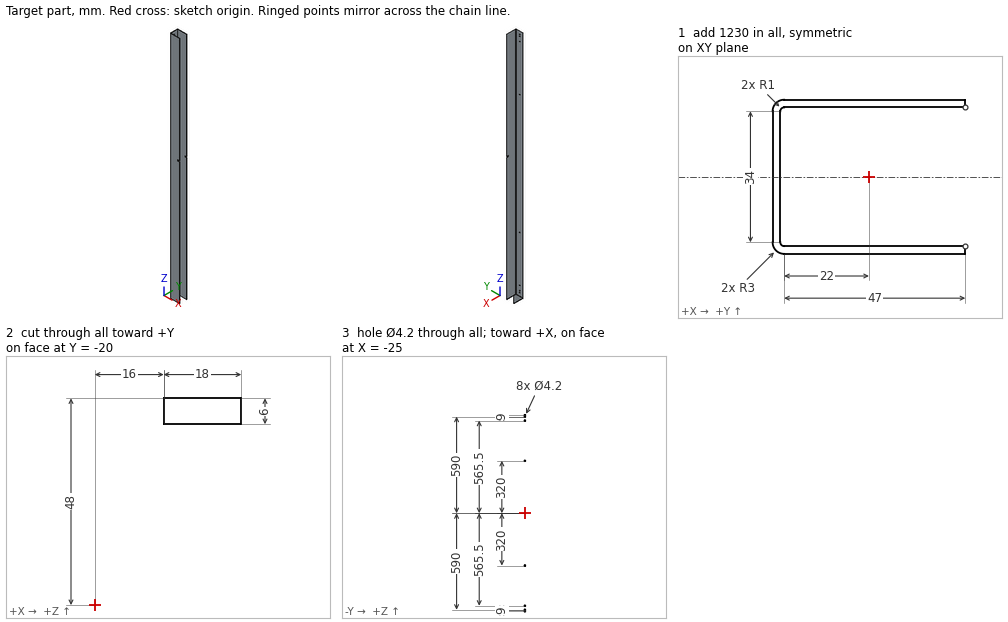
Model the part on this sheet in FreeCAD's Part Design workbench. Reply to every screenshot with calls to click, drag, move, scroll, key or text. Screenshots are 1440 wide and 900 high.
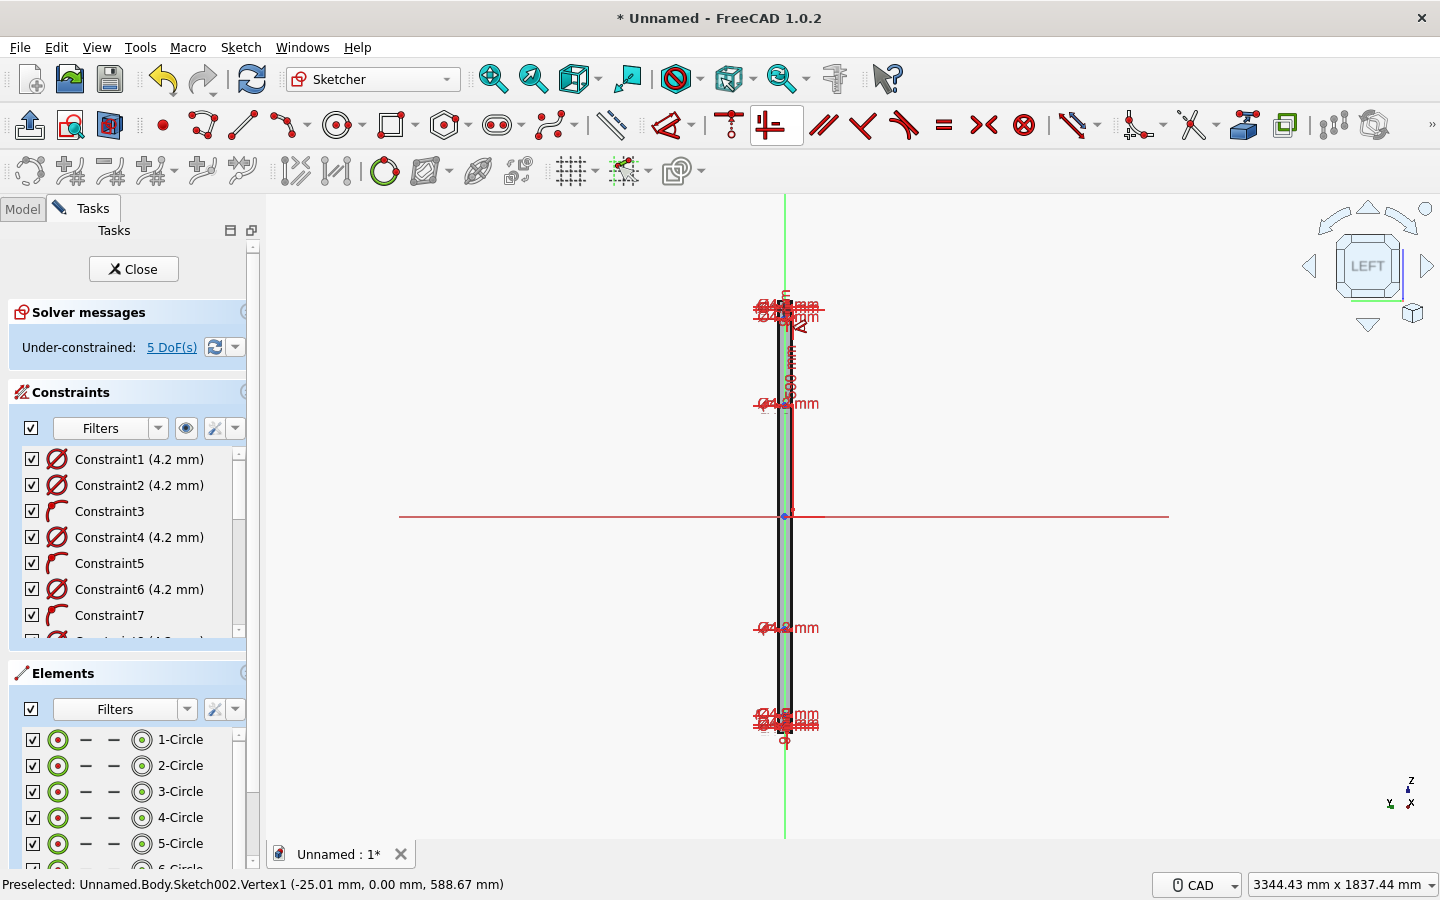
click(785, 406)
click(819, 461)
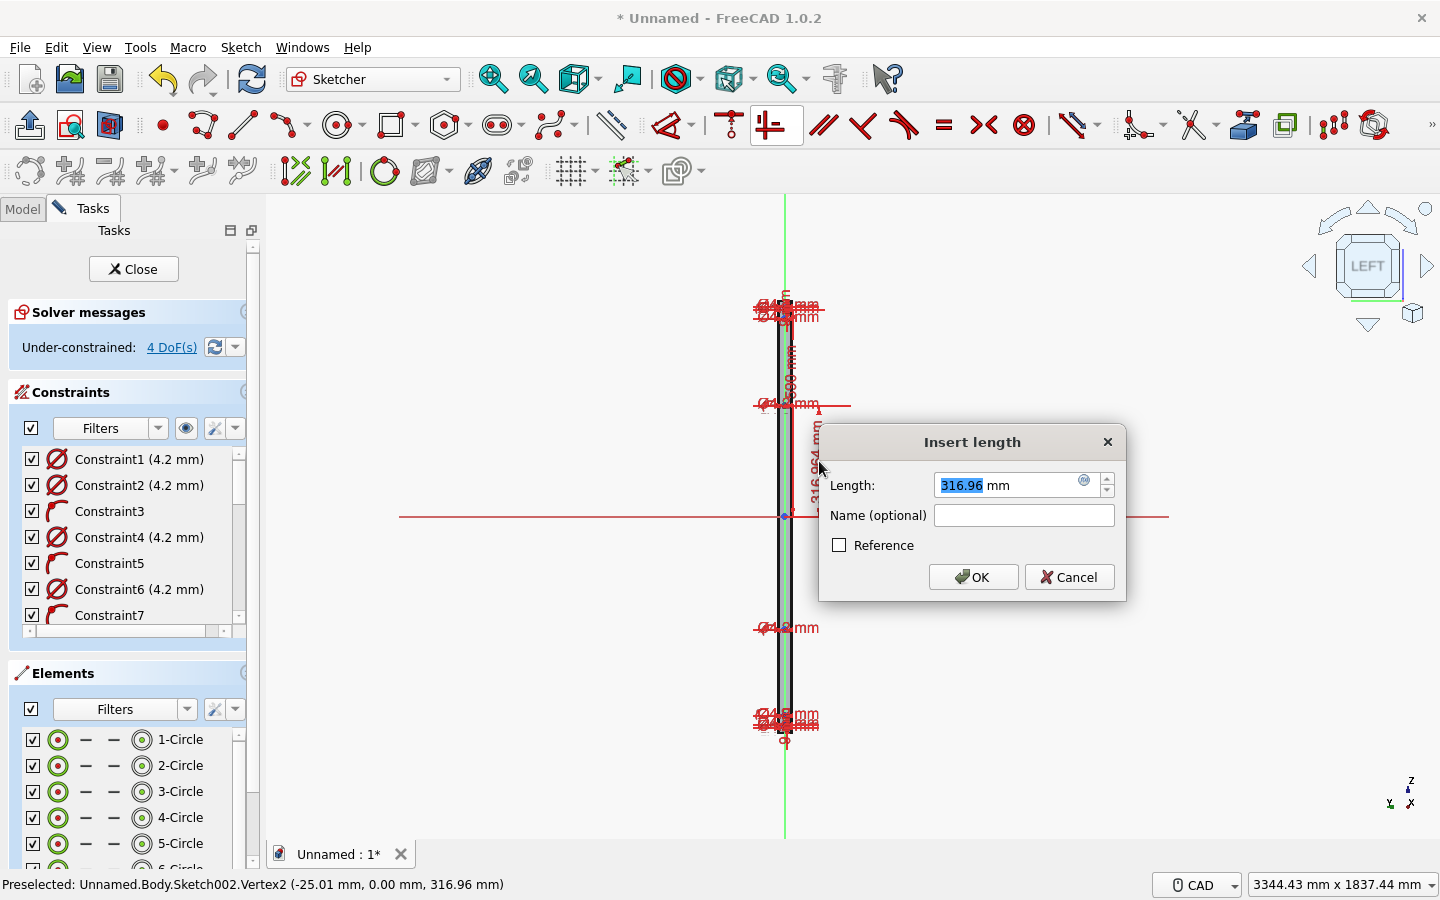
text(320)
key(Return)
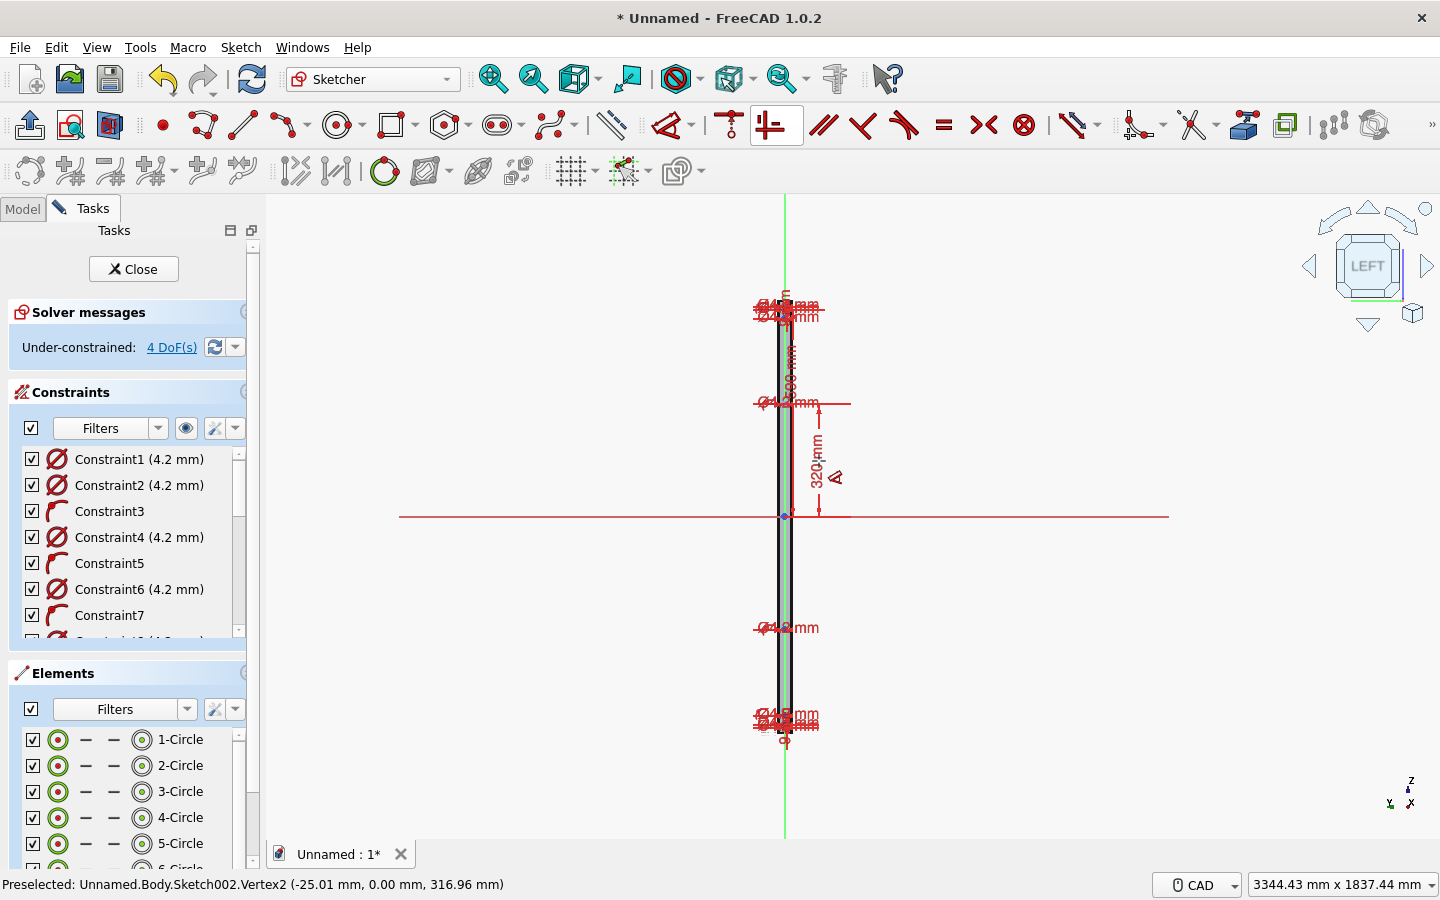
click(785, 630)
click(819, 573)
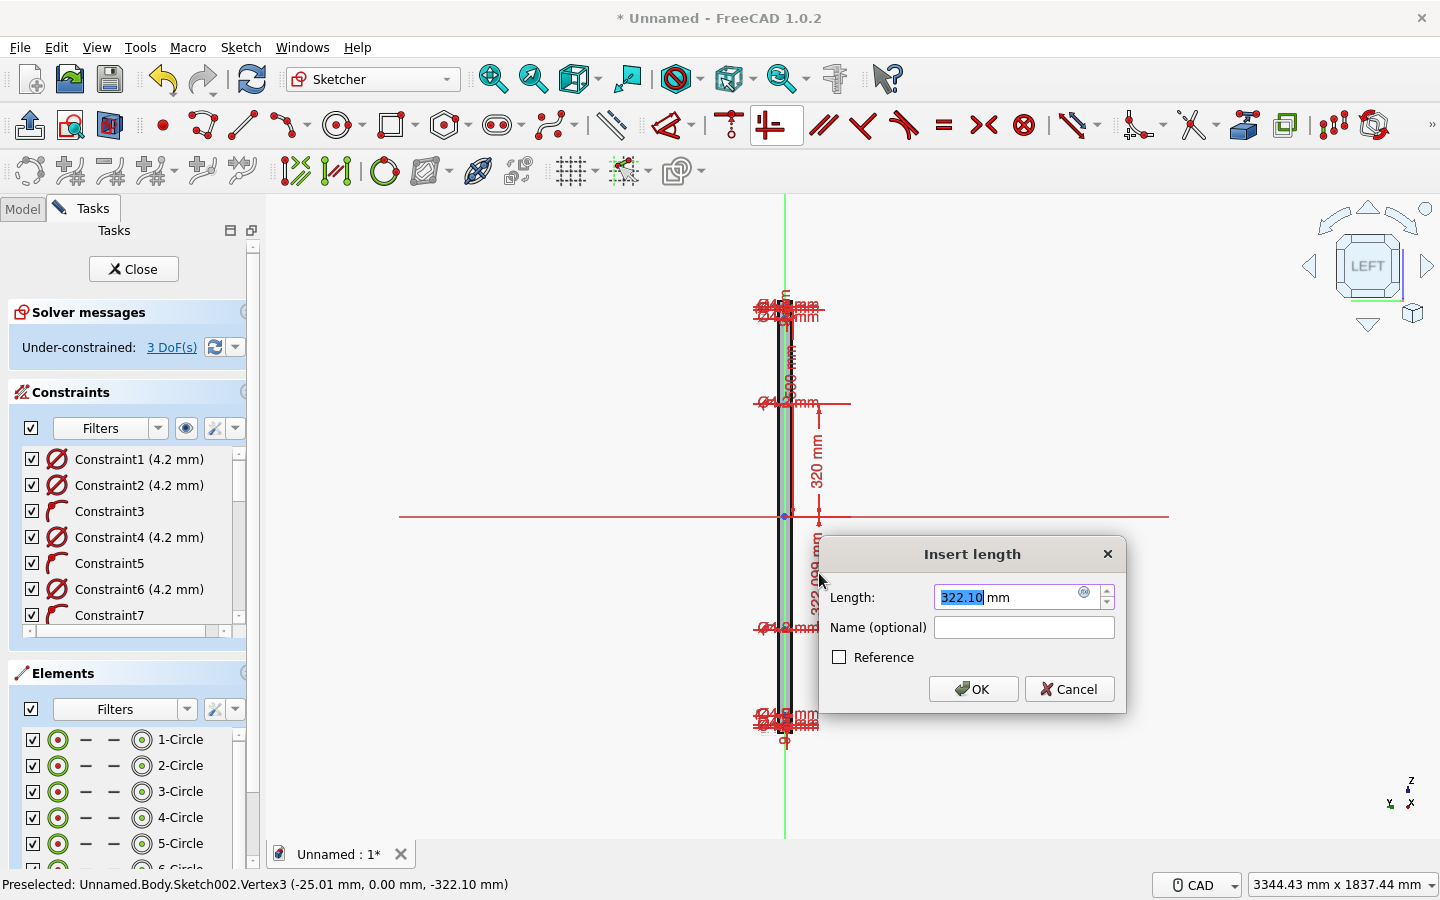
text(320)
key(Return)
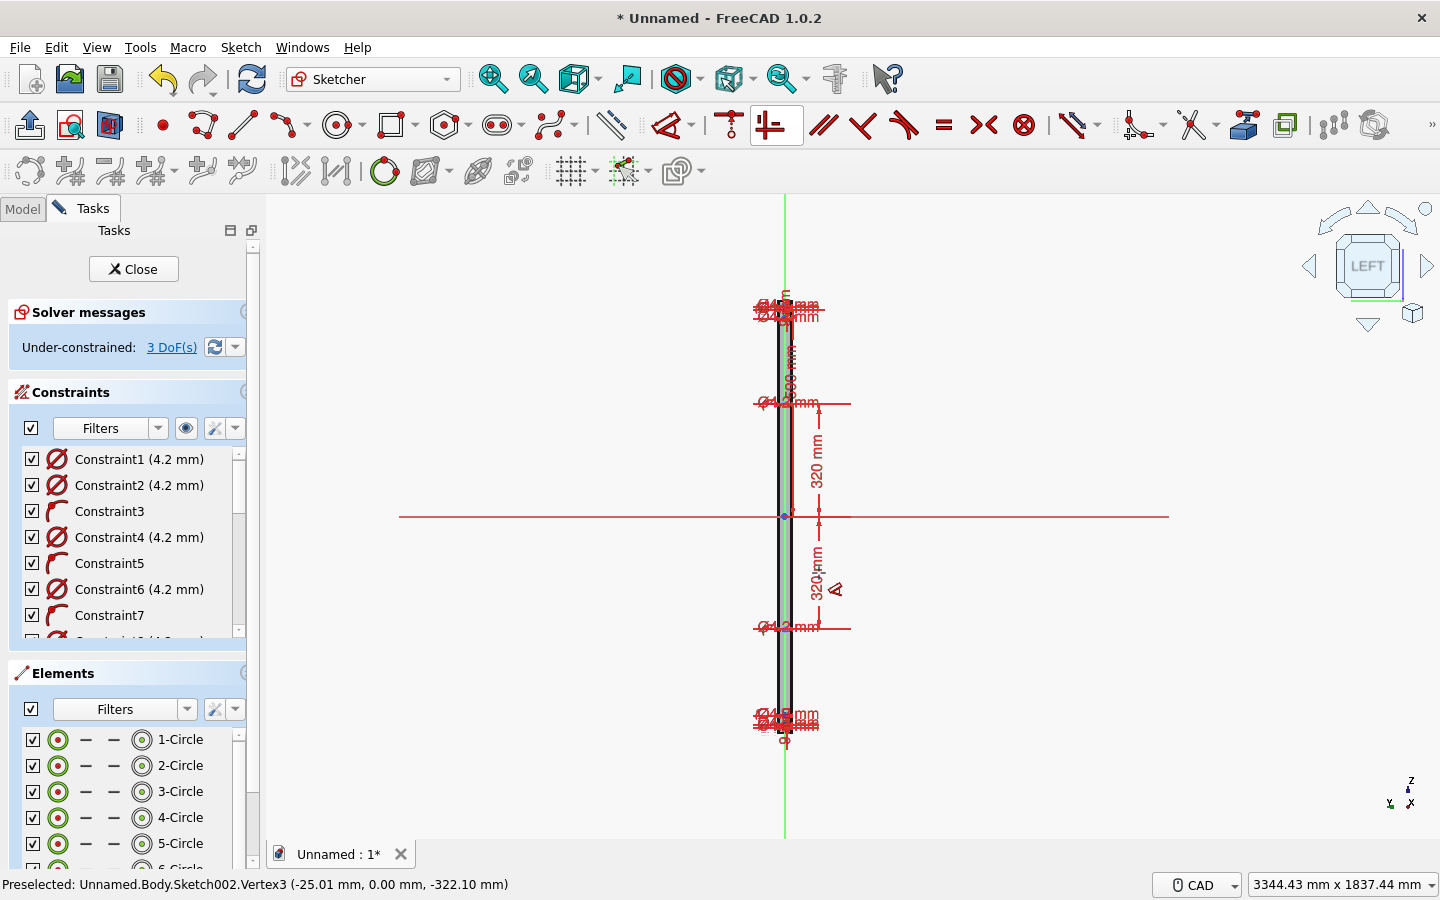
scroll(785, 725, up, 7)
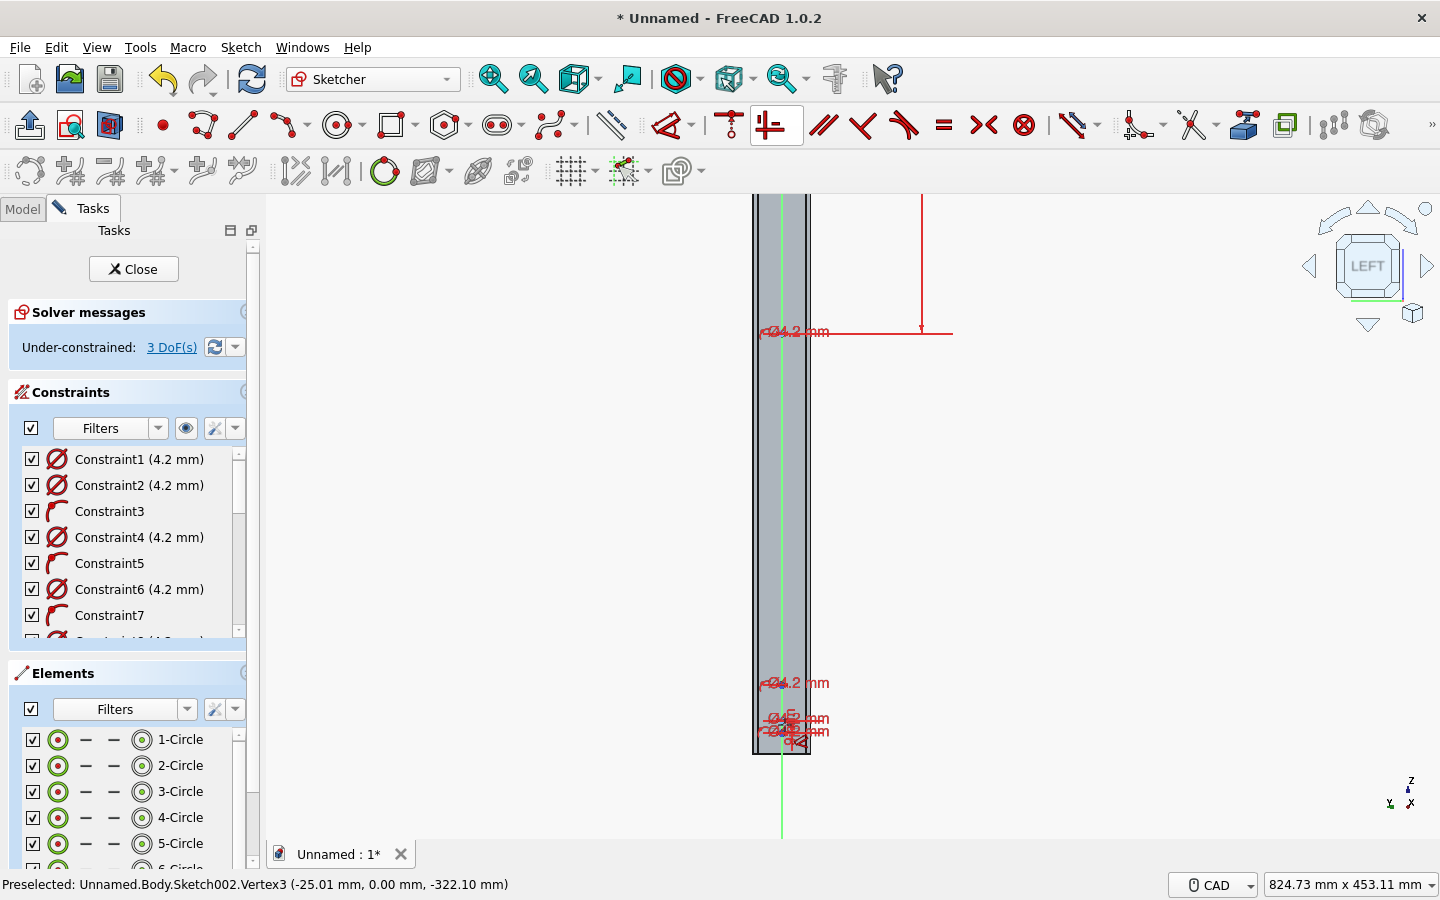
click(782, 721)
click(816, 471)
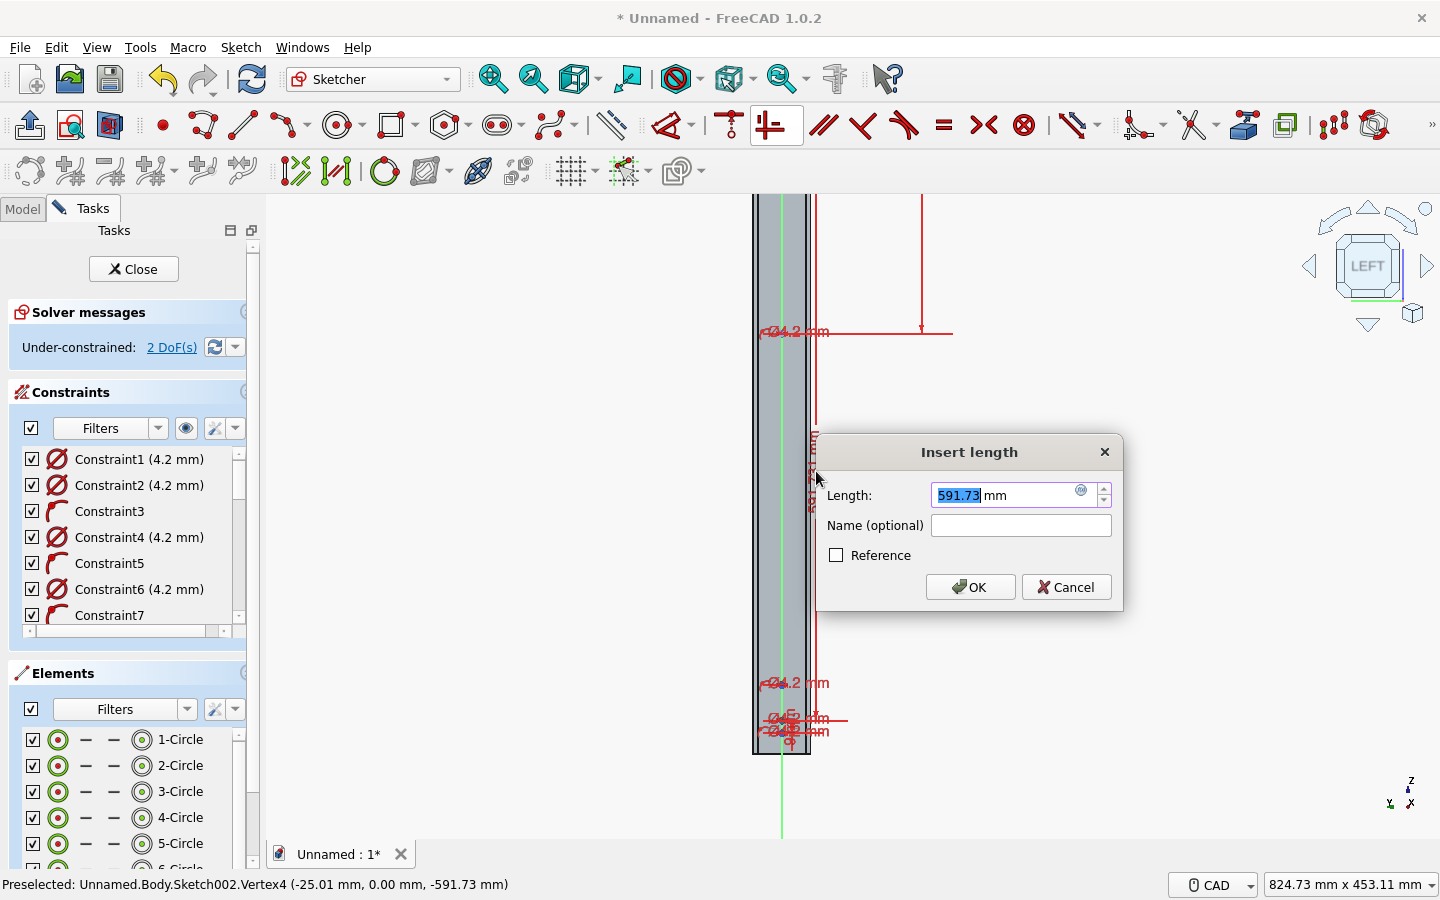
text(590)
key(Return)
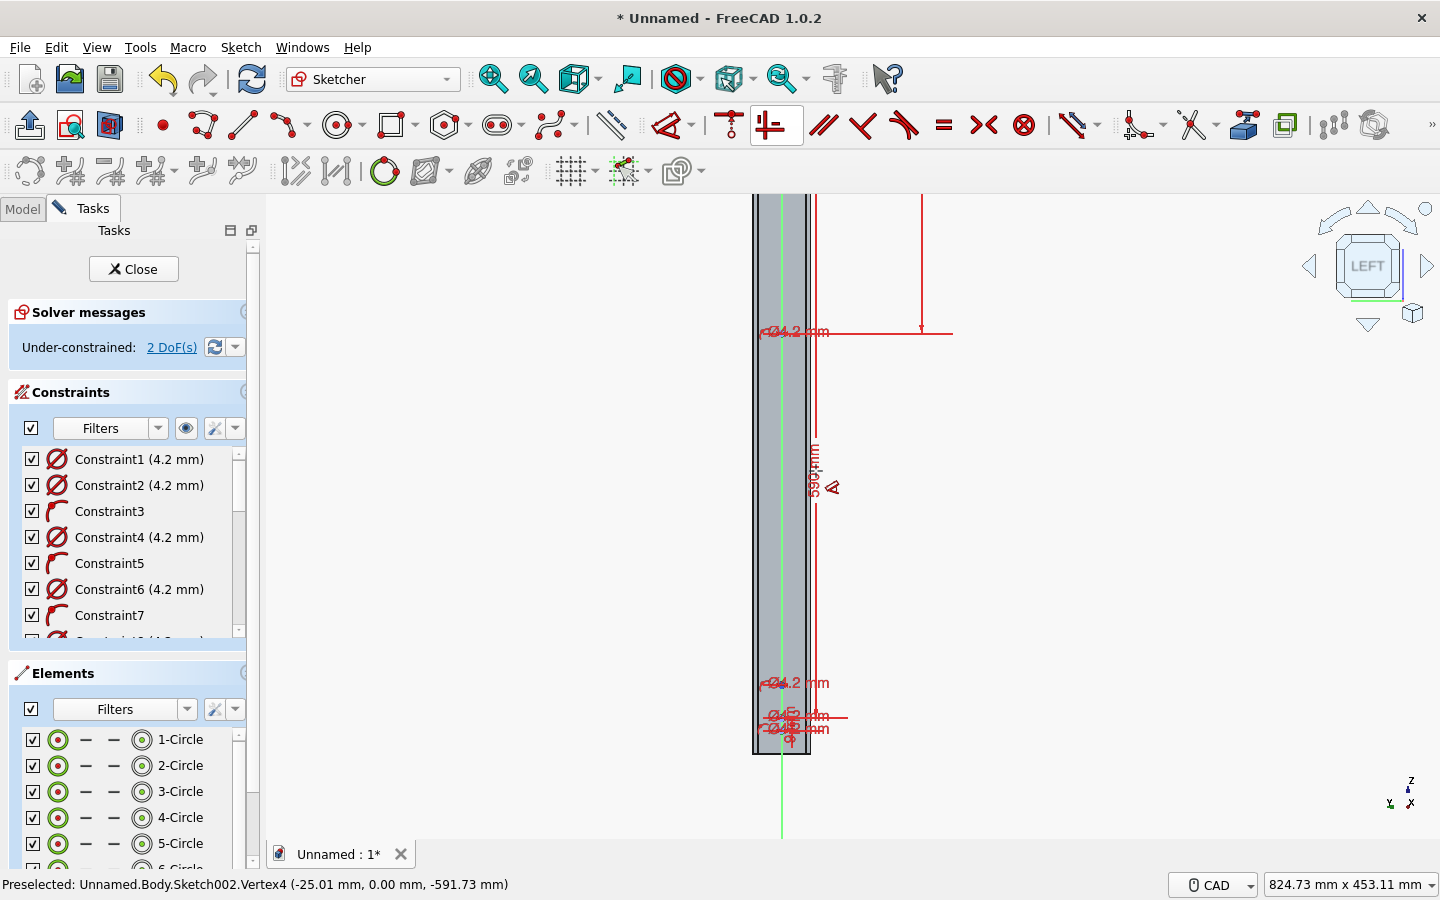
scroll(785, 725, down, 7)